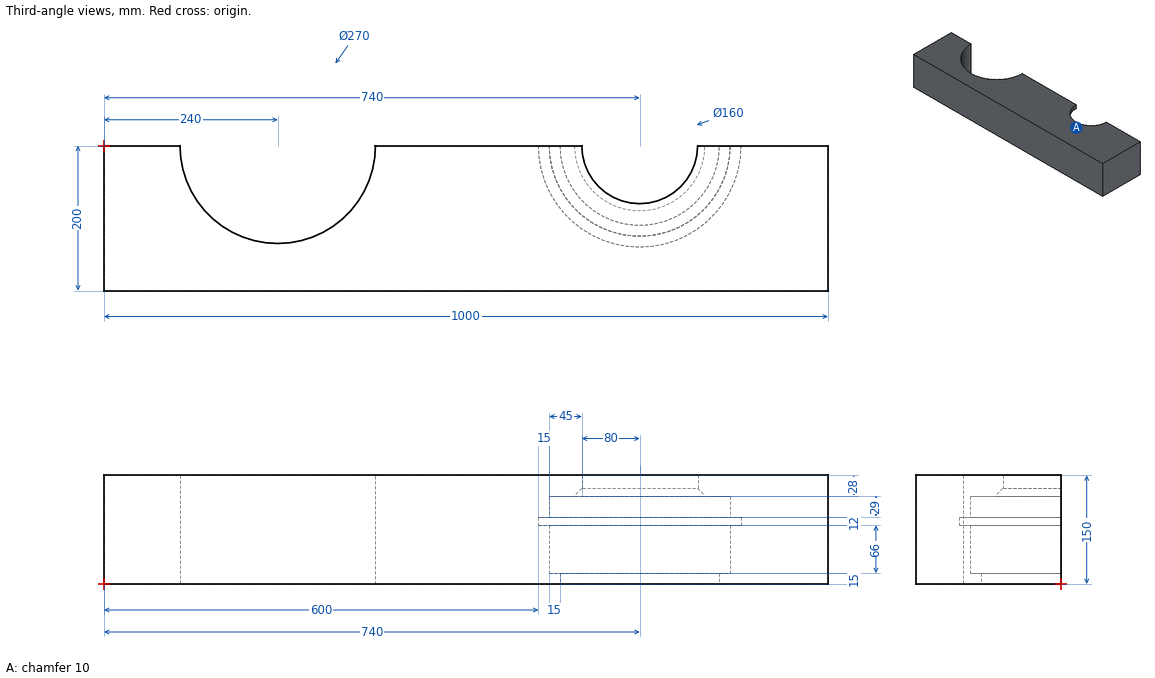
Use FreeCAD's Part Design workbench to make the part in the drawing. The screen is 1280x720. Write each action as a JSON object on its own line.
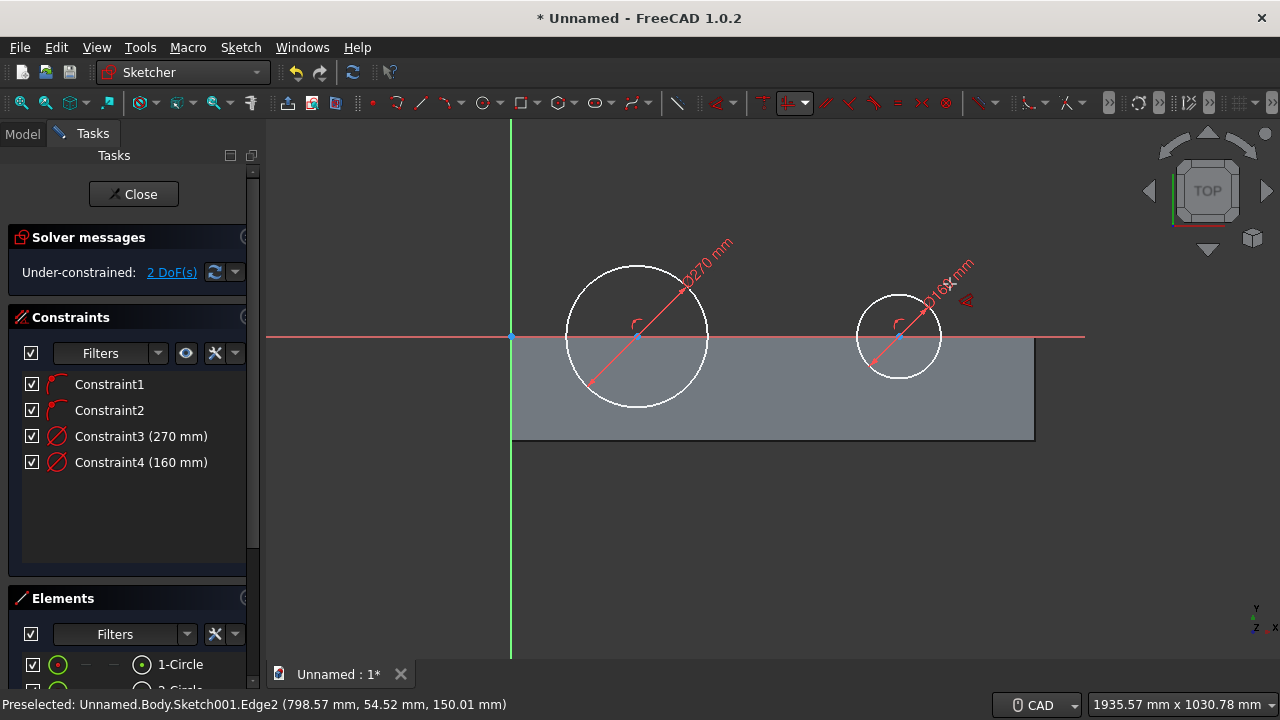
{"action": "left_click", "coordinate": [637, 337]}
{"action": "left_click", "coordinate": [545, 371]}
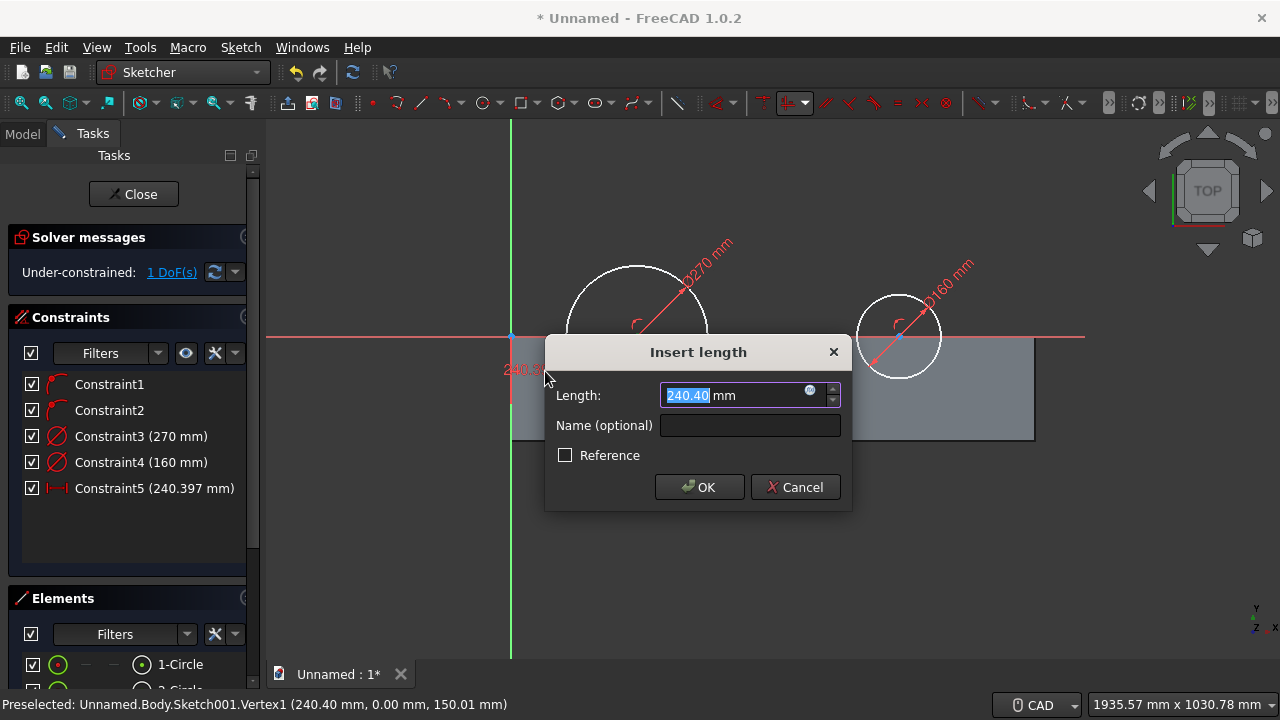
{"action": "type", "text": "240"}
{"action": "key", "text": "Return"}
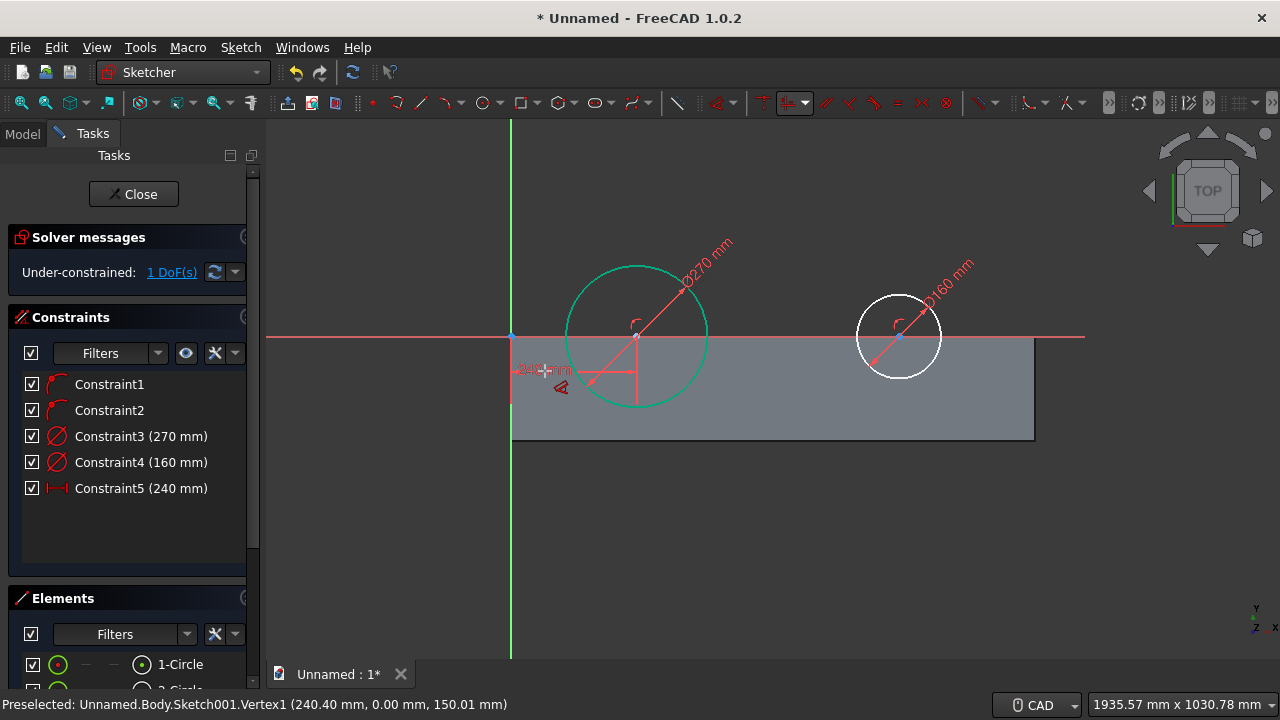
{"action": "left_click", "coordinate": [899, 337]}
{"action": "left_click", "coordinate": [616, 371]}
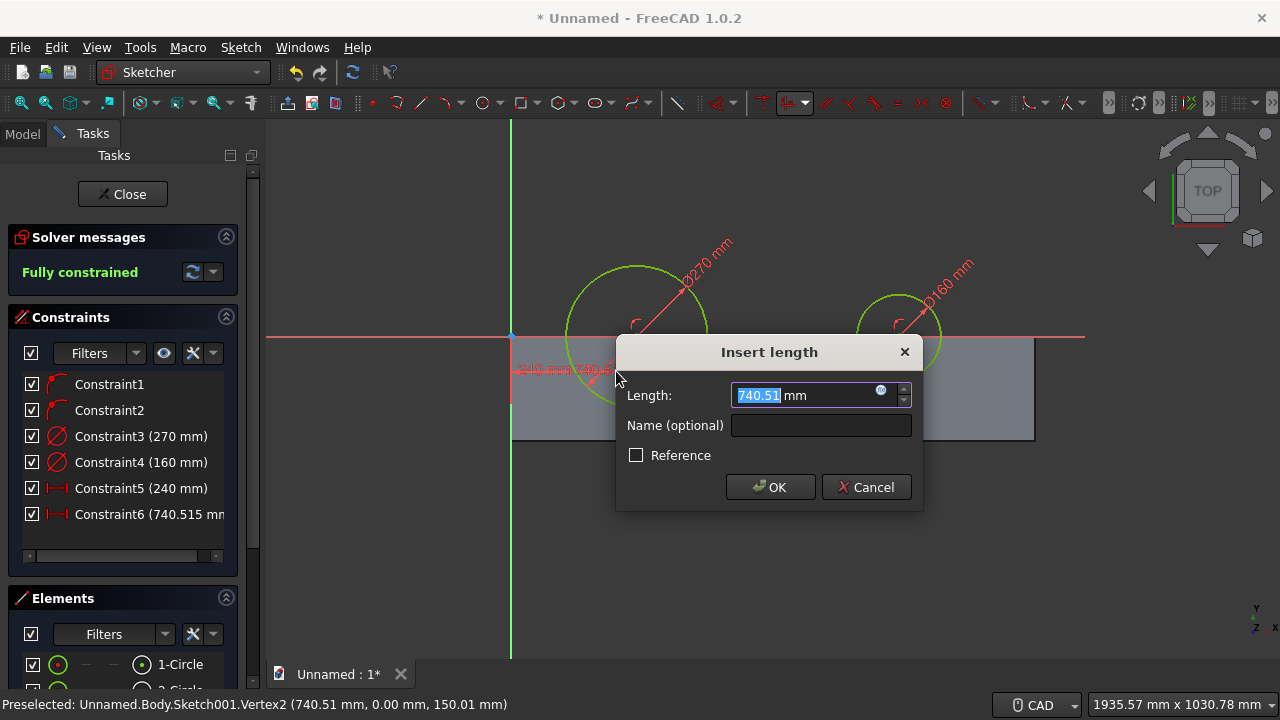
{"action": "type", "text": "740"}
{"action": "key", "text": "Return"}
{"action": "key", "text": "Escape"}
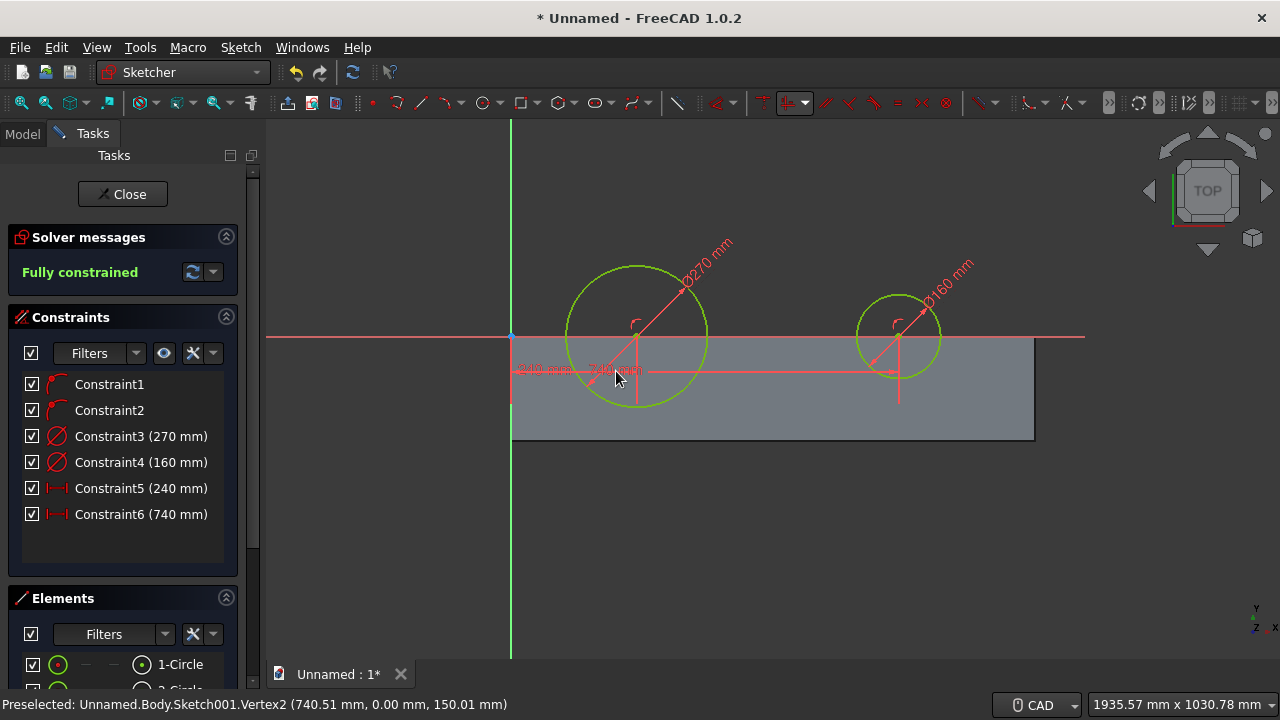
{"action": "left_click", "coordinate": [123, 194]}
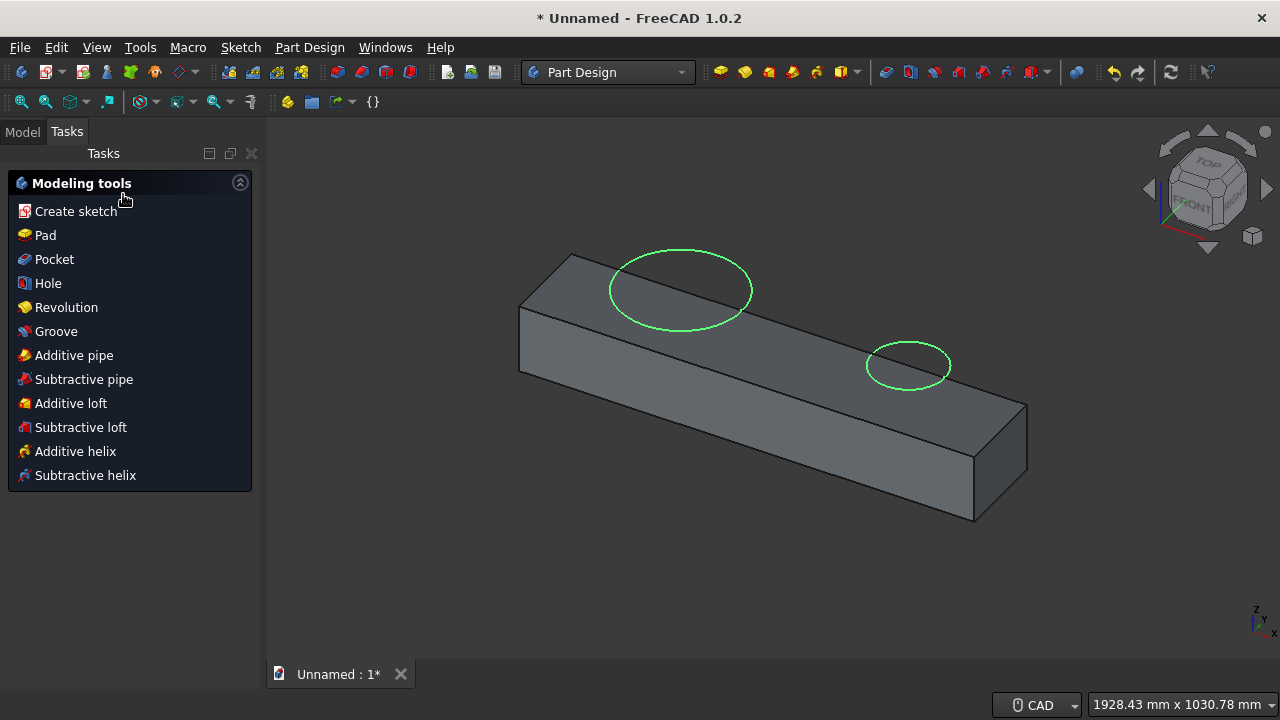
{"action": "left_click", "coordinate": [888, 72]}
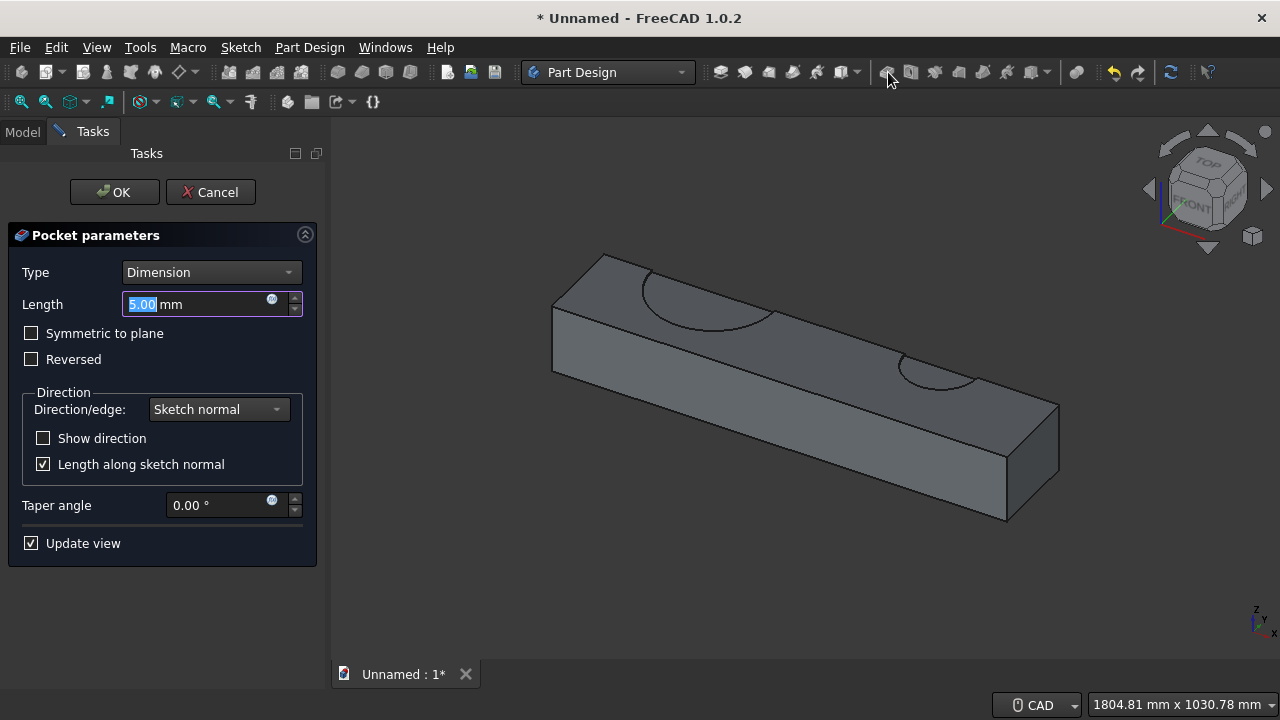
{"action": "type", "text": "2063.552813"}
{"action": "key", "text": "Tab"}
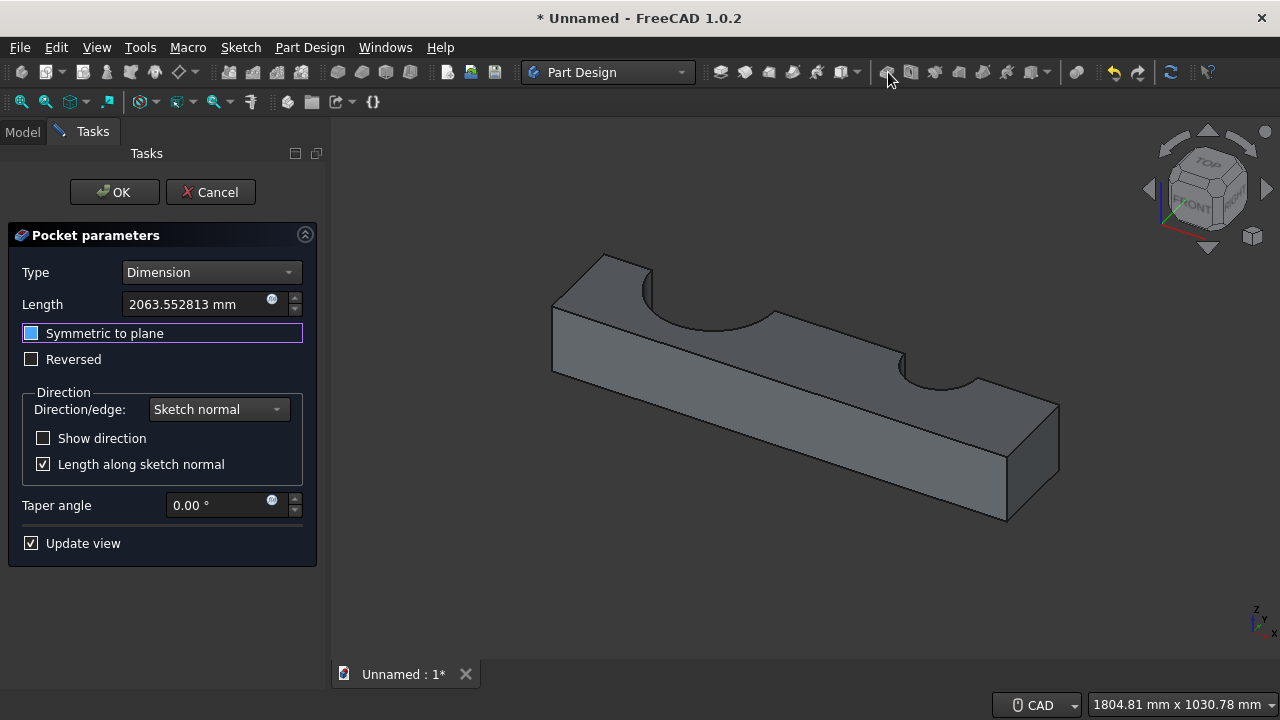
{"action": "left_click", "coordinate": [30, 333]}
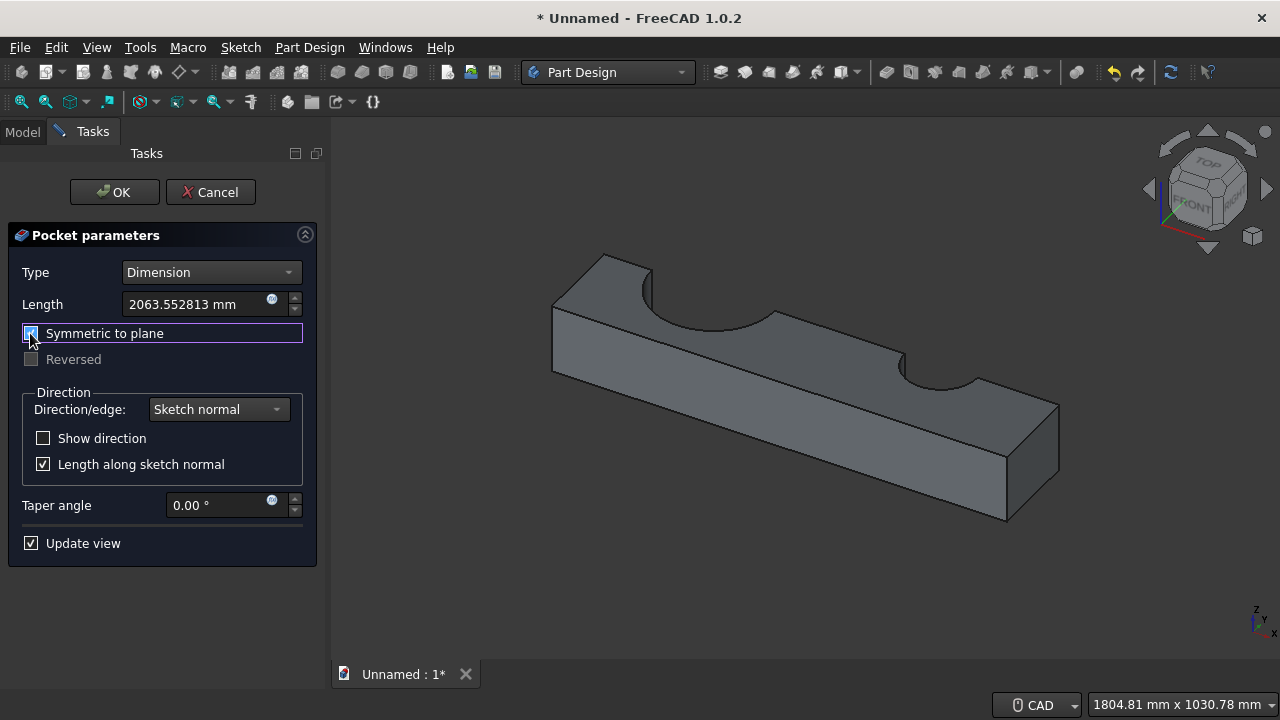
{"action": "left_click", "coordinate": [115, 192]}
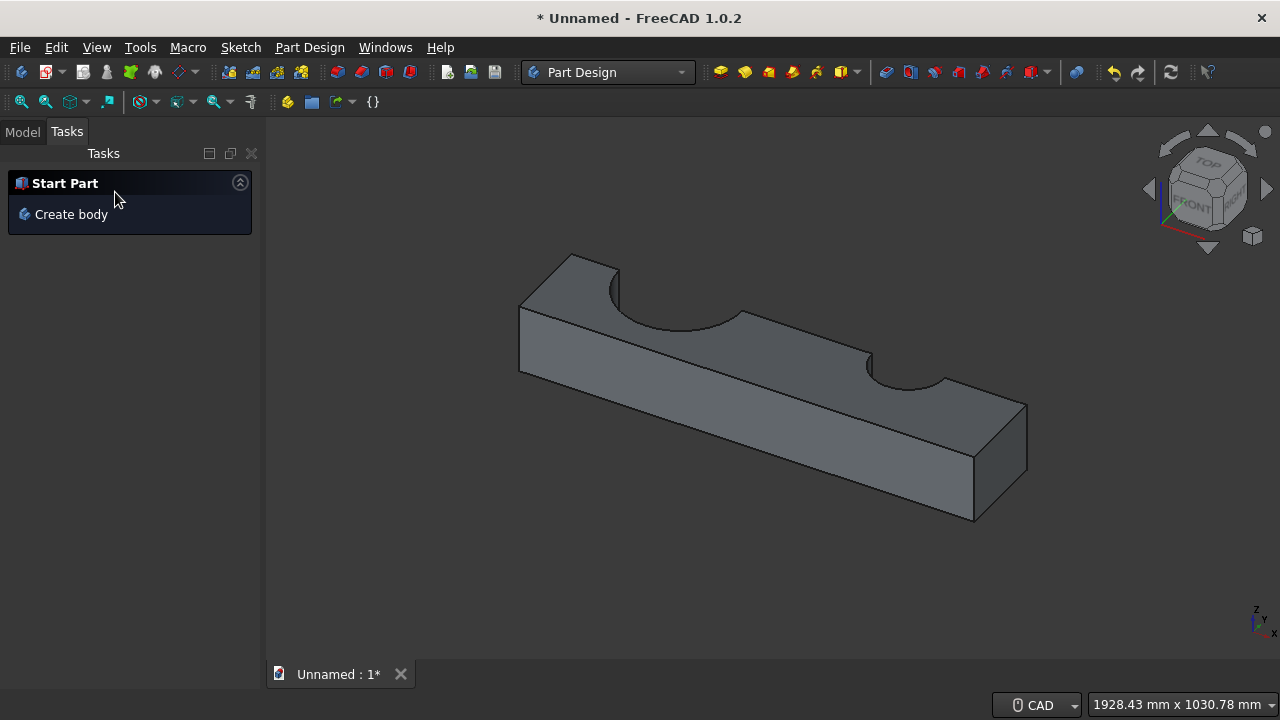
{"action": "key", "text": "4"}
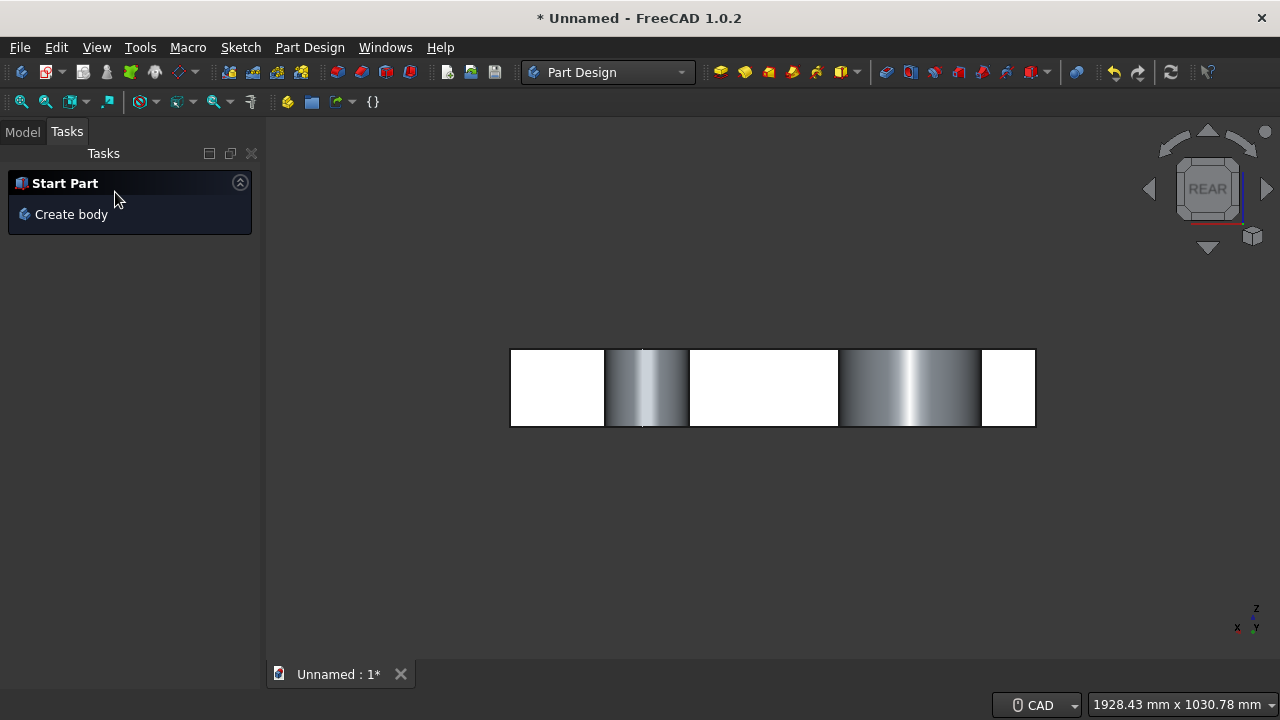
{"action": "left_click", "coordinate": [742, 387]}